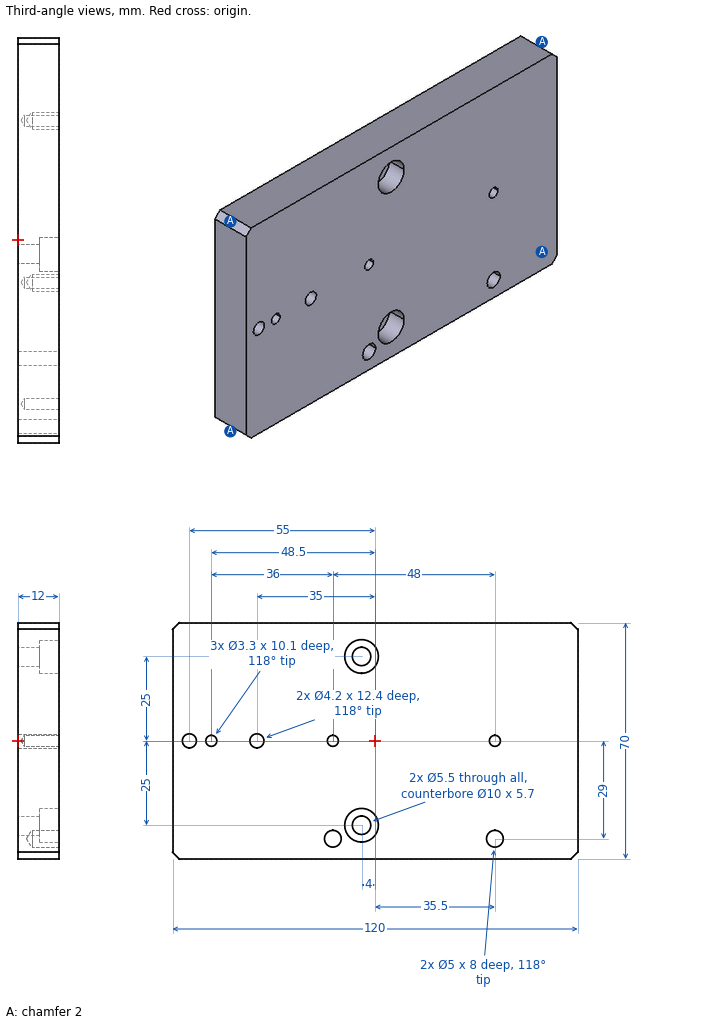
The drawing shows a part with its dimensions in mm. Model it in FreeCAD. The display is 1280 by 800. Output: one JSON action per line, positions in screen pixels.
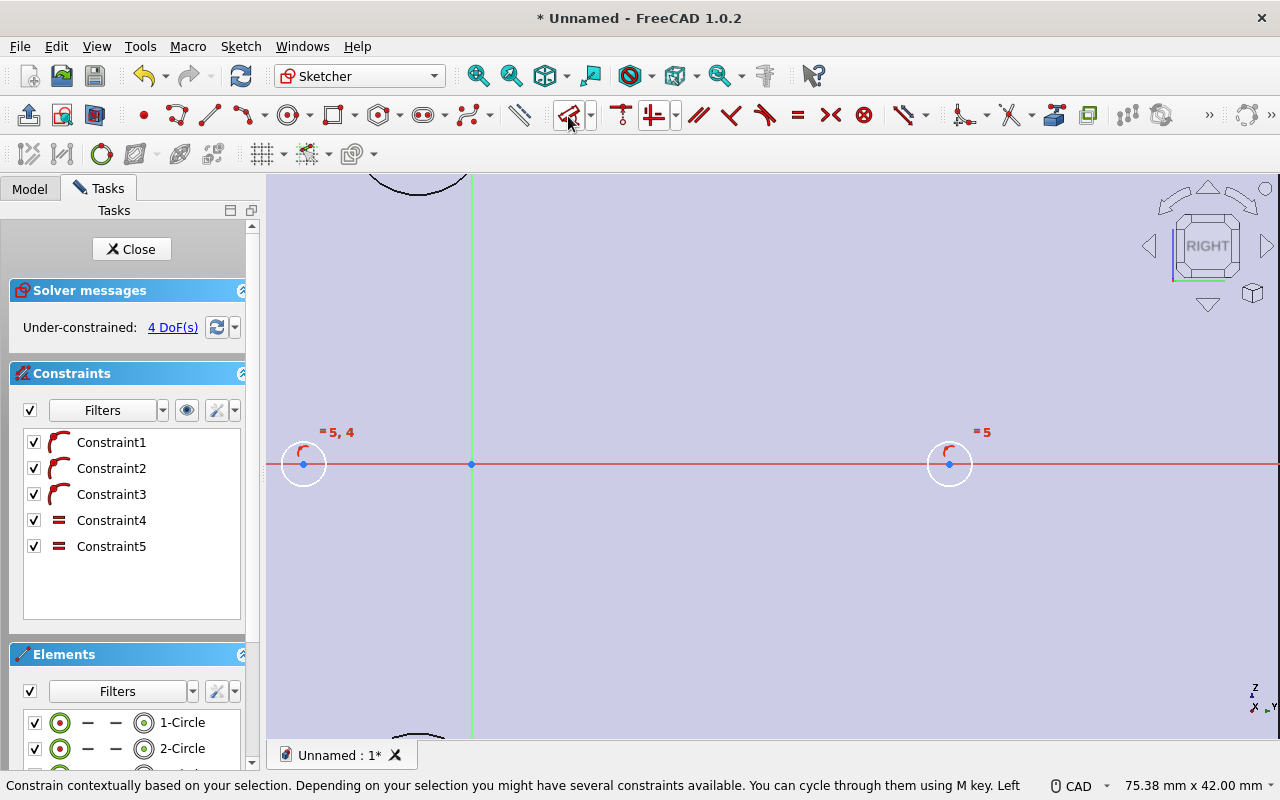
{"action": "scroll", "coordinate": [966, 450], "scroll_direction": "down", "scroll_amount": 4}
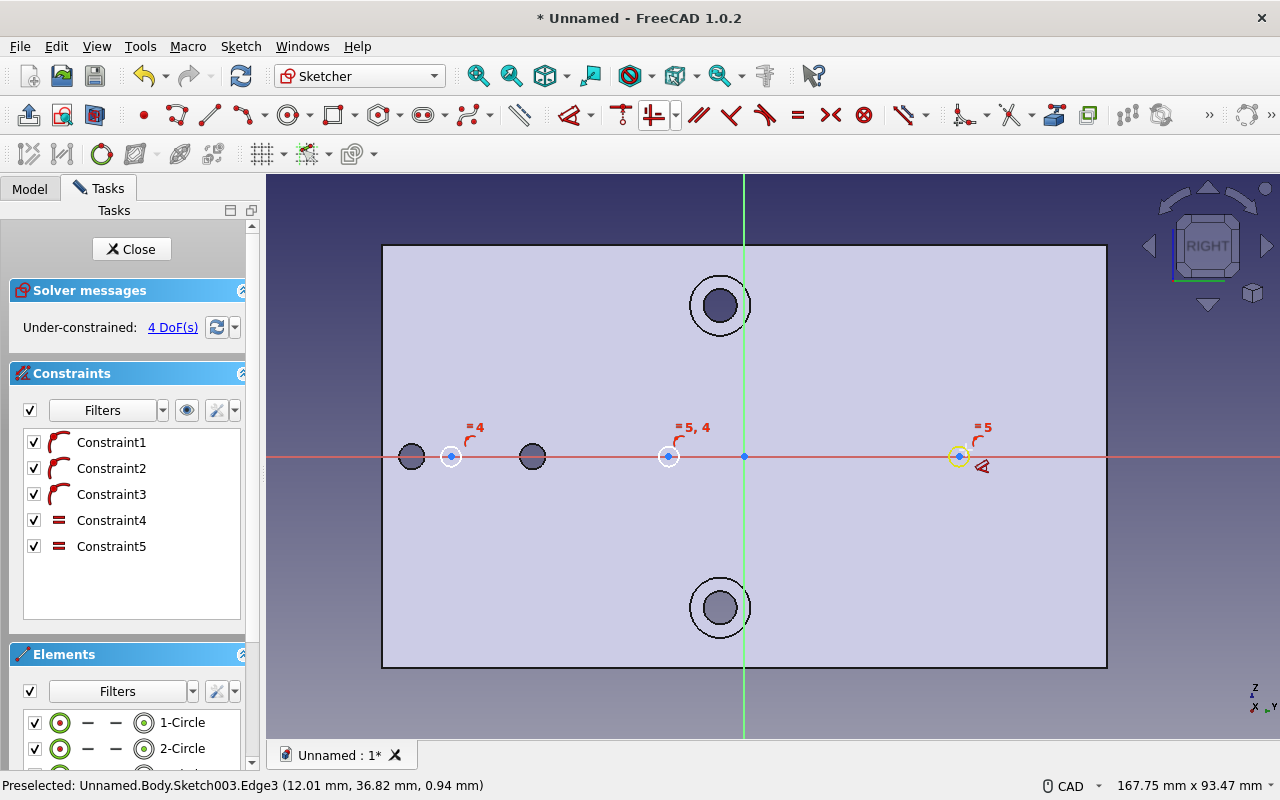
{"action": "scroll", "coordinate": [458, 450], "scroll_direction": "up", "scroll_amount": 4}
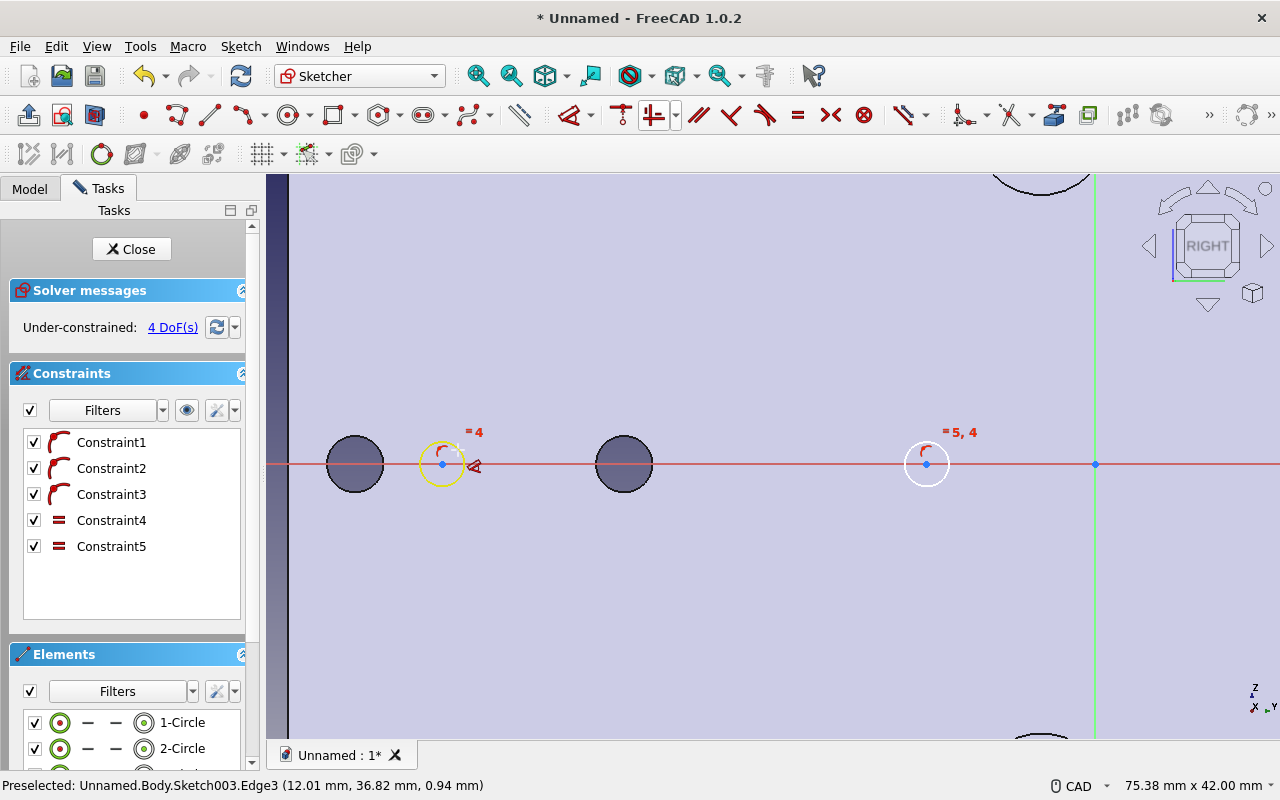
{"action": "left_click", "coordinate": [458, 448]}
{"action": "left_click", "coordinate": [480, 425]}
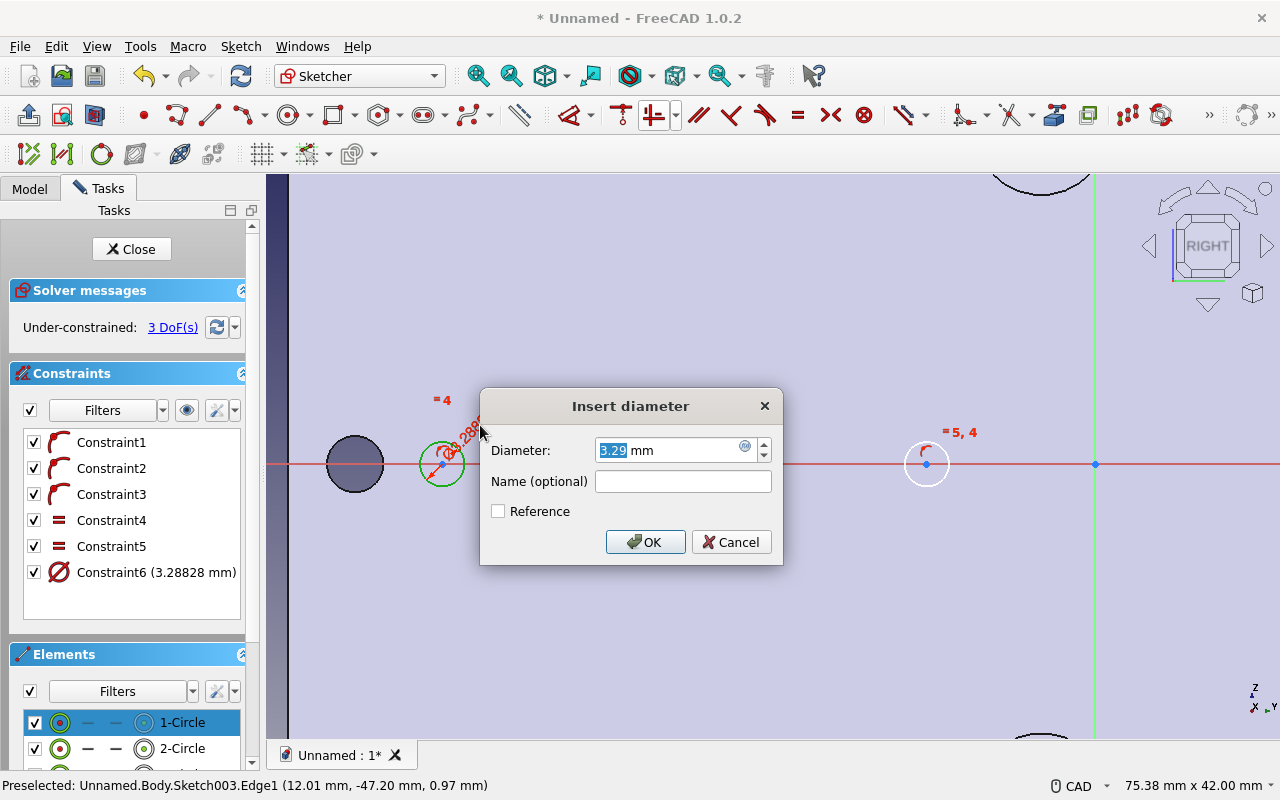
{"action": "type", "text": "3.3"}
{"action": "key", "text": "Return"}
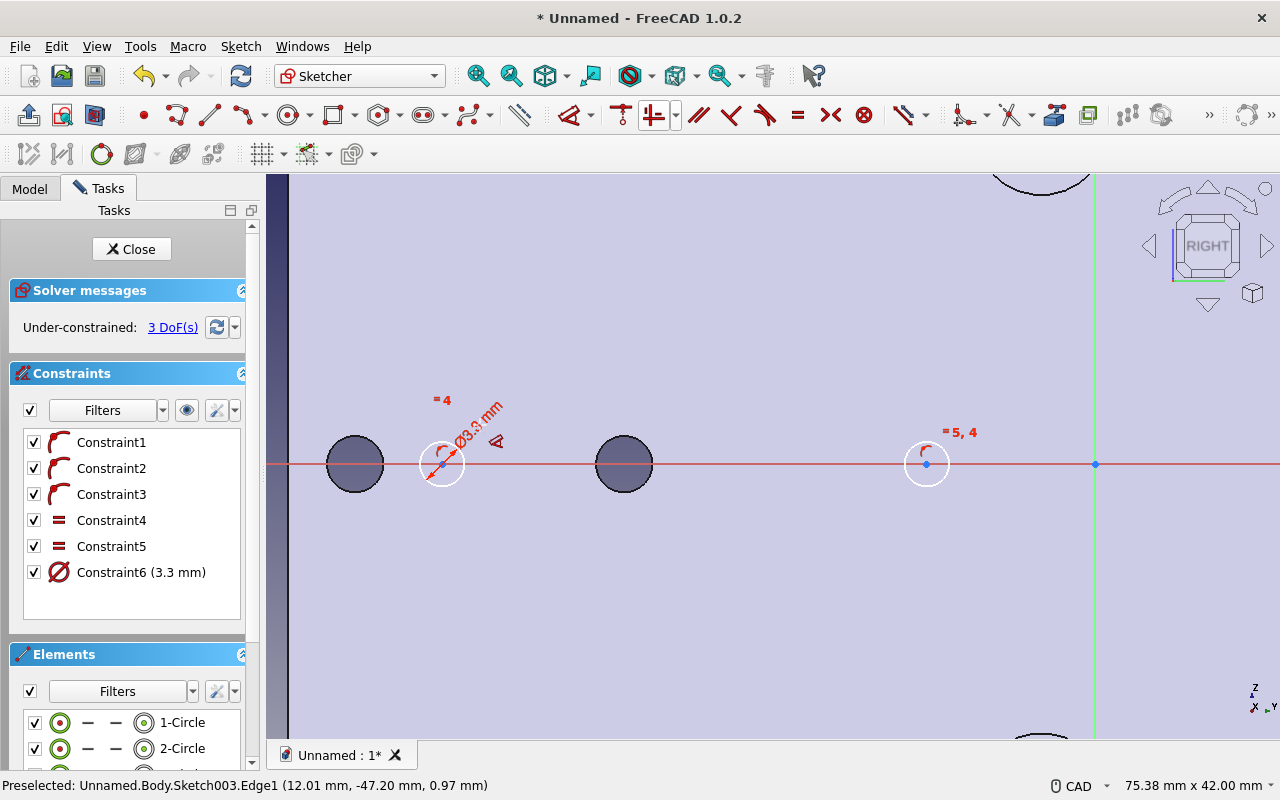
{"action": "left_click", "coordinate": [442, 464]}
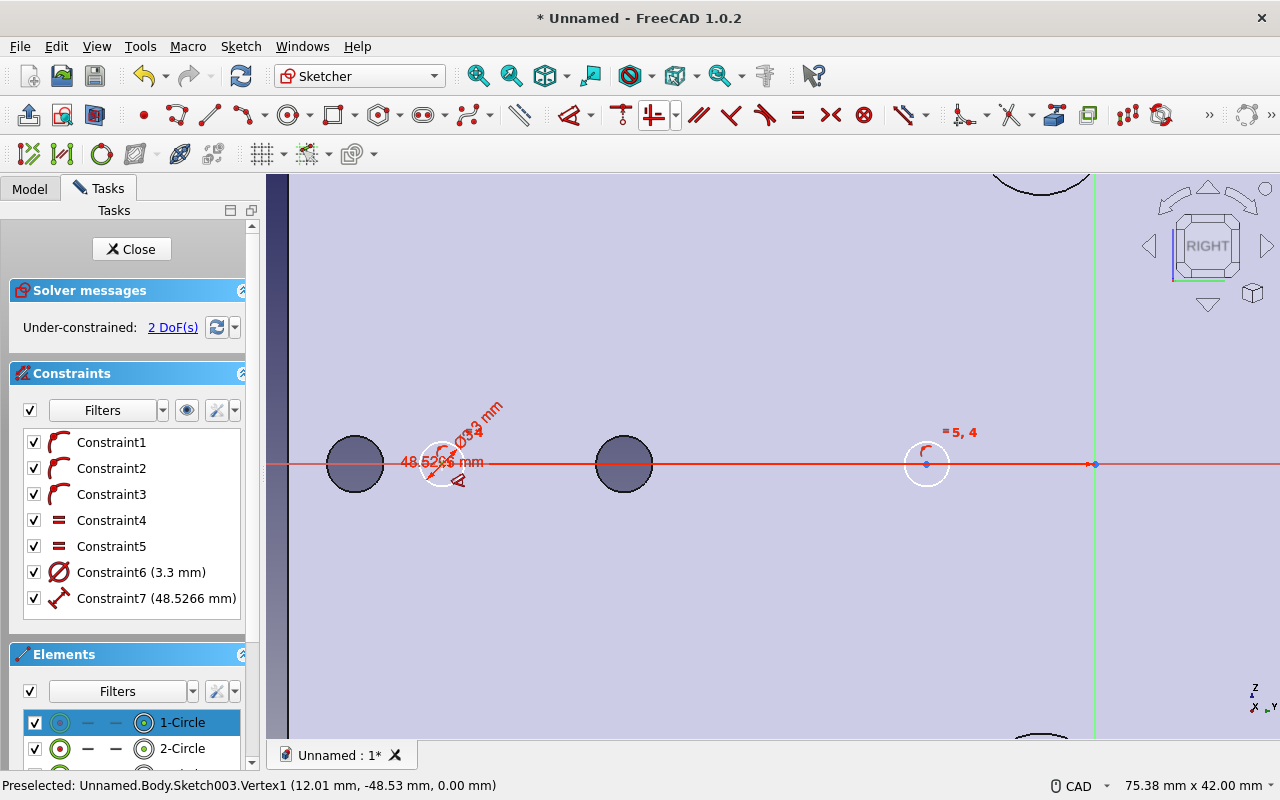
{"action": "left_click", "coordinate": [927, 464]}
{"action": "left_click", "coordinate": [685, 498]}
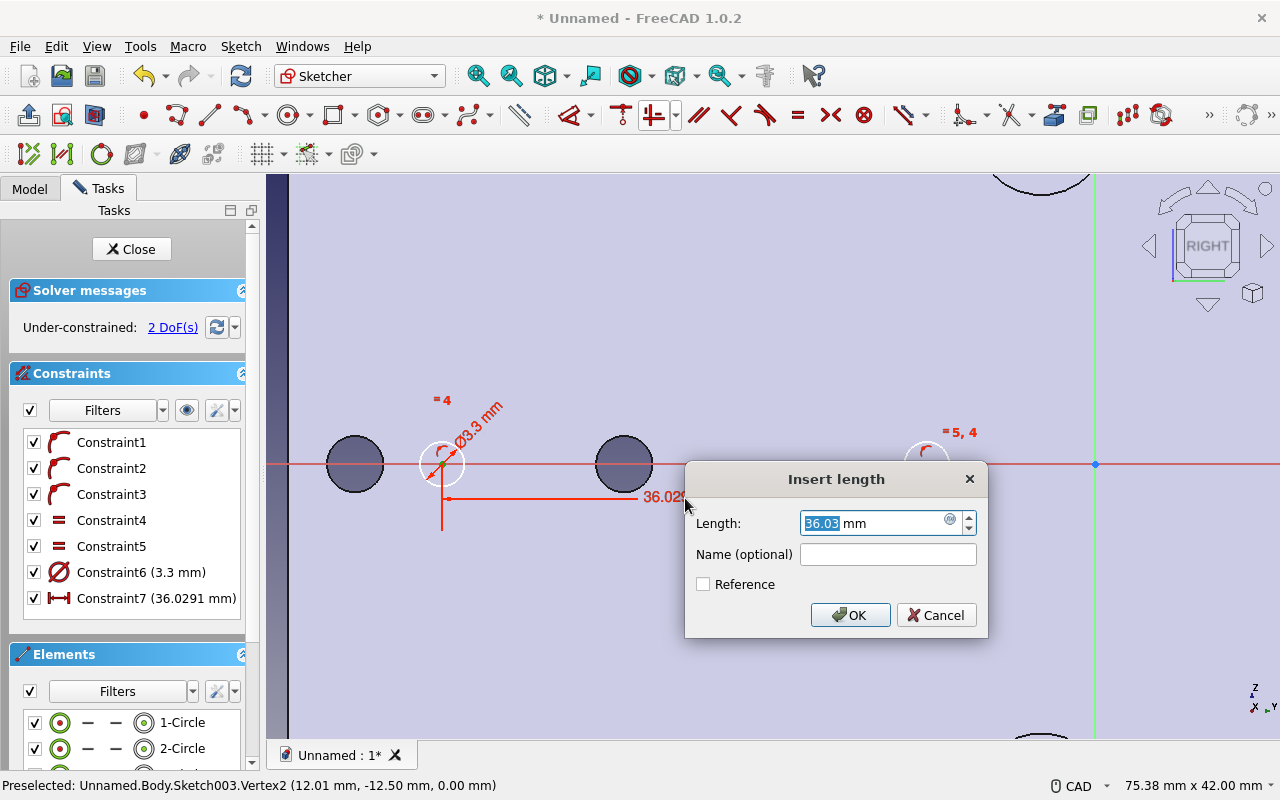
{"action": "type", "text": "36"}
{"action": "key", "text": "Return"}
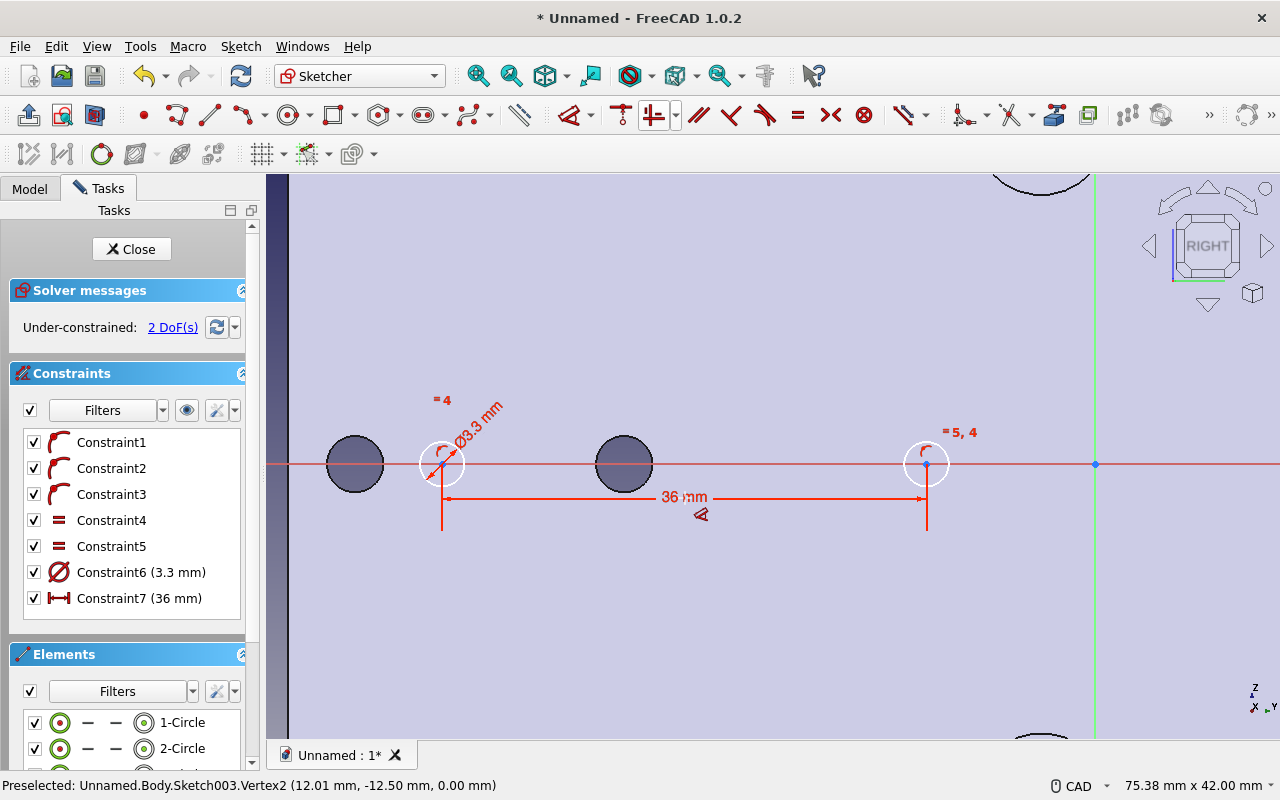
{"action": "left_click", "coordinate": [927, 464]}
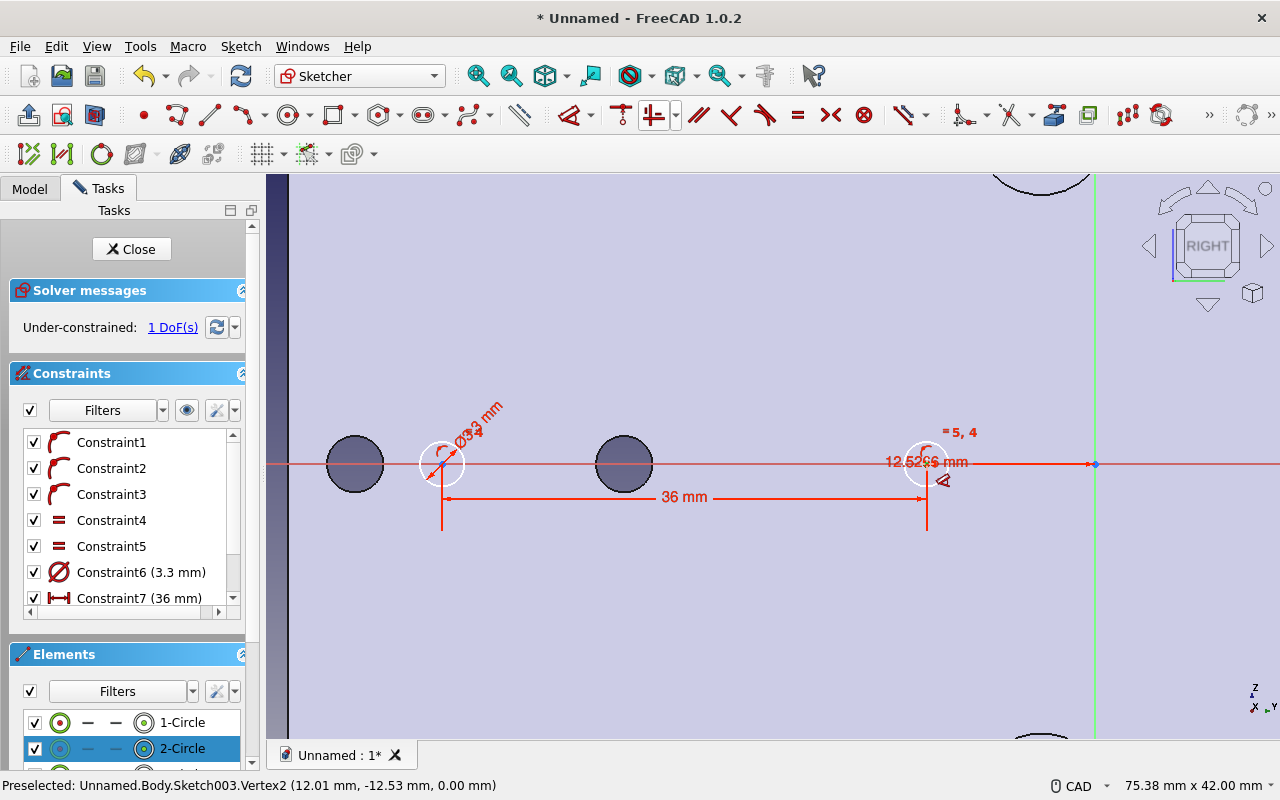
{"action": "scroll", "coordinate": [457, 450], "scroll_direction": "down", "scroll_amount": 4}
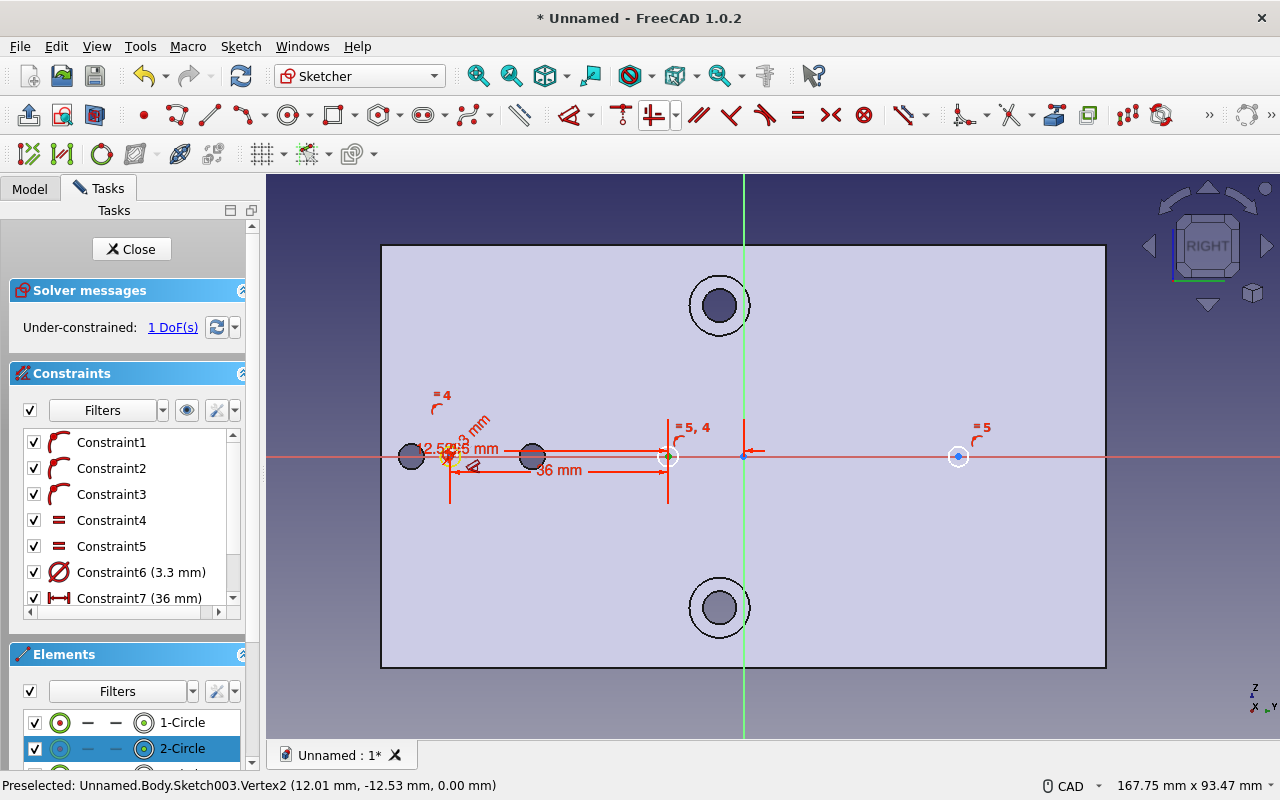
{"action": "left_click", "coordinate": [959, 457]}
{"action": "left_click", "coordinate": [813, 491]}